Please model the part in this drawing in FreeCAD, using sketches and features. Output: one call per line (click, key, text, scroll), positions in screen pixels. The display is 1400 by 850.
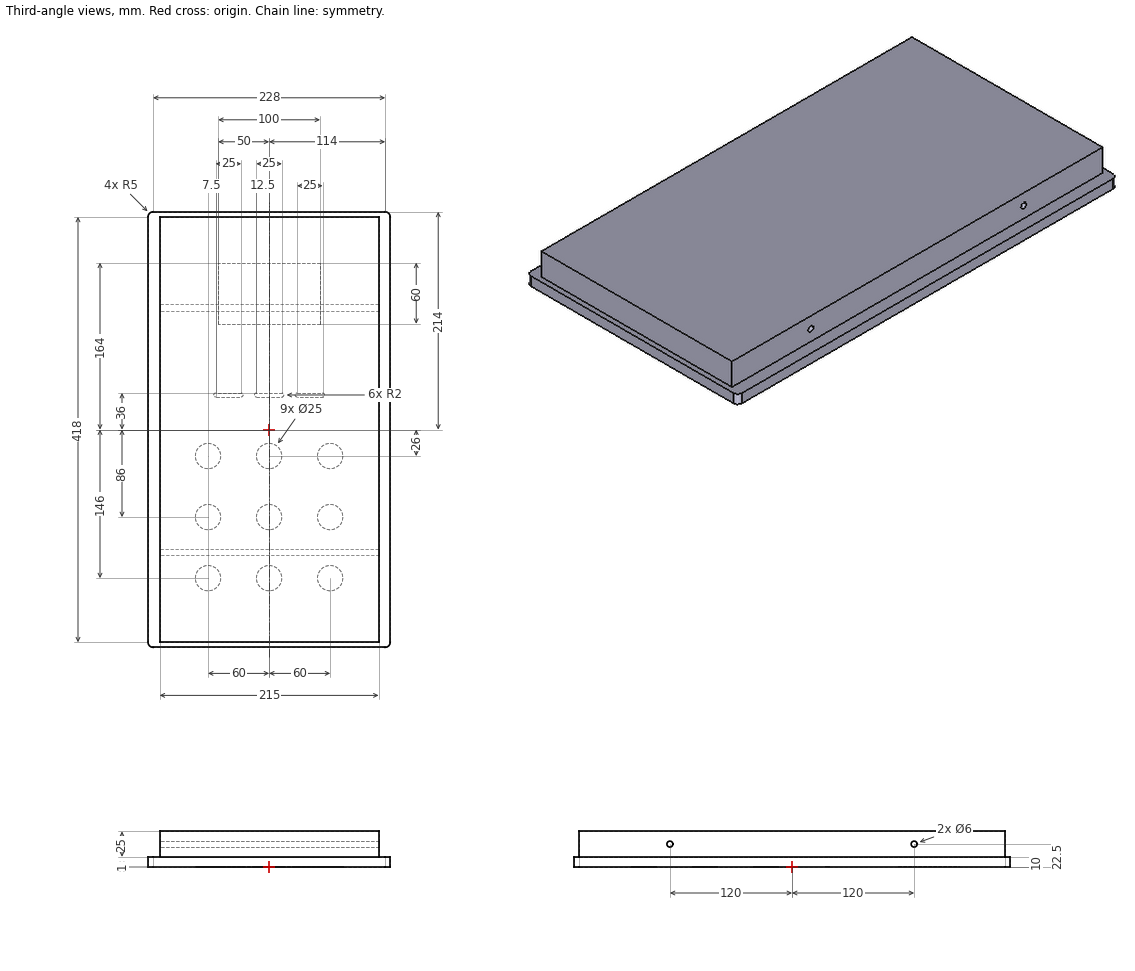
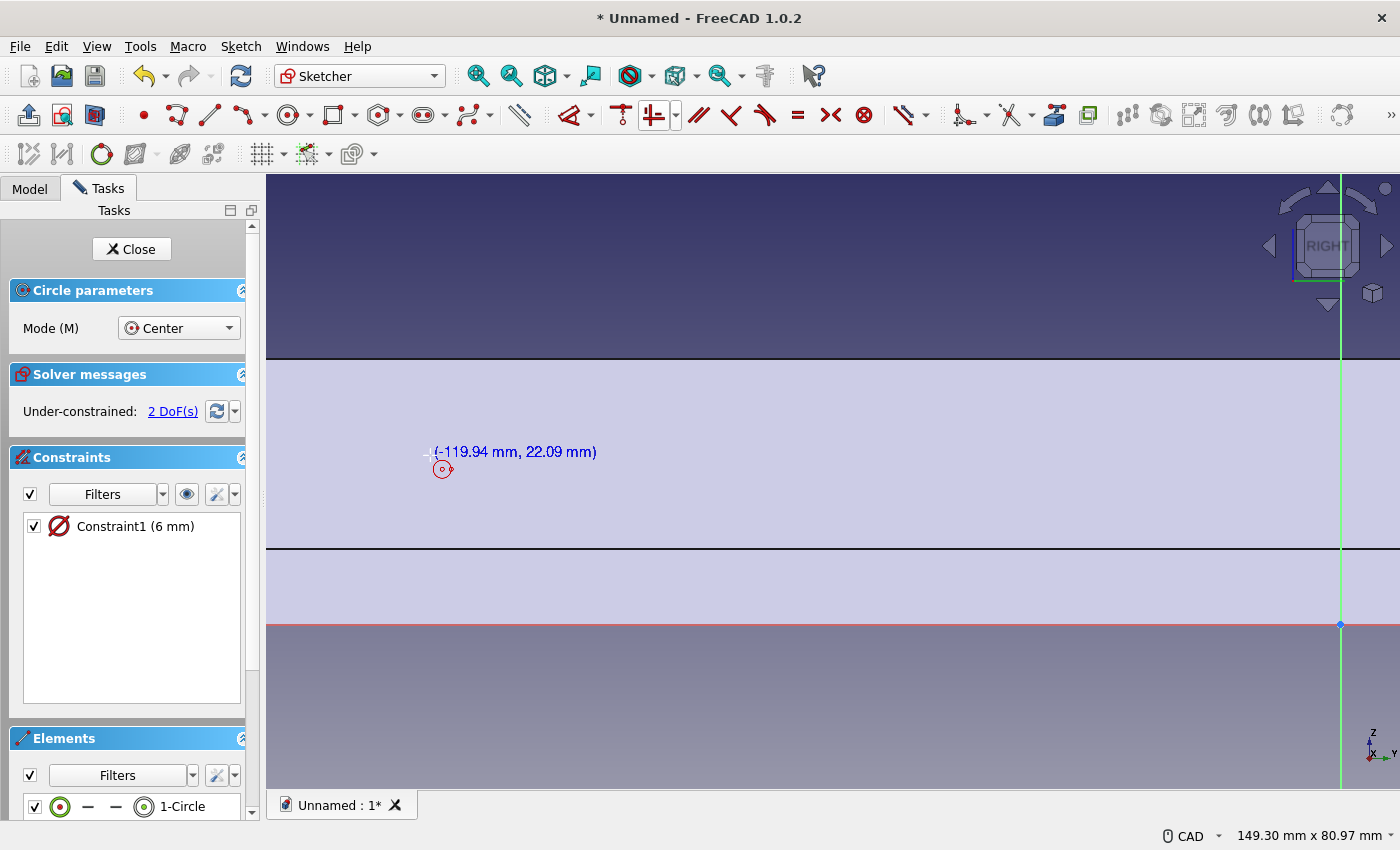
click(429, 454)
move(445, 438)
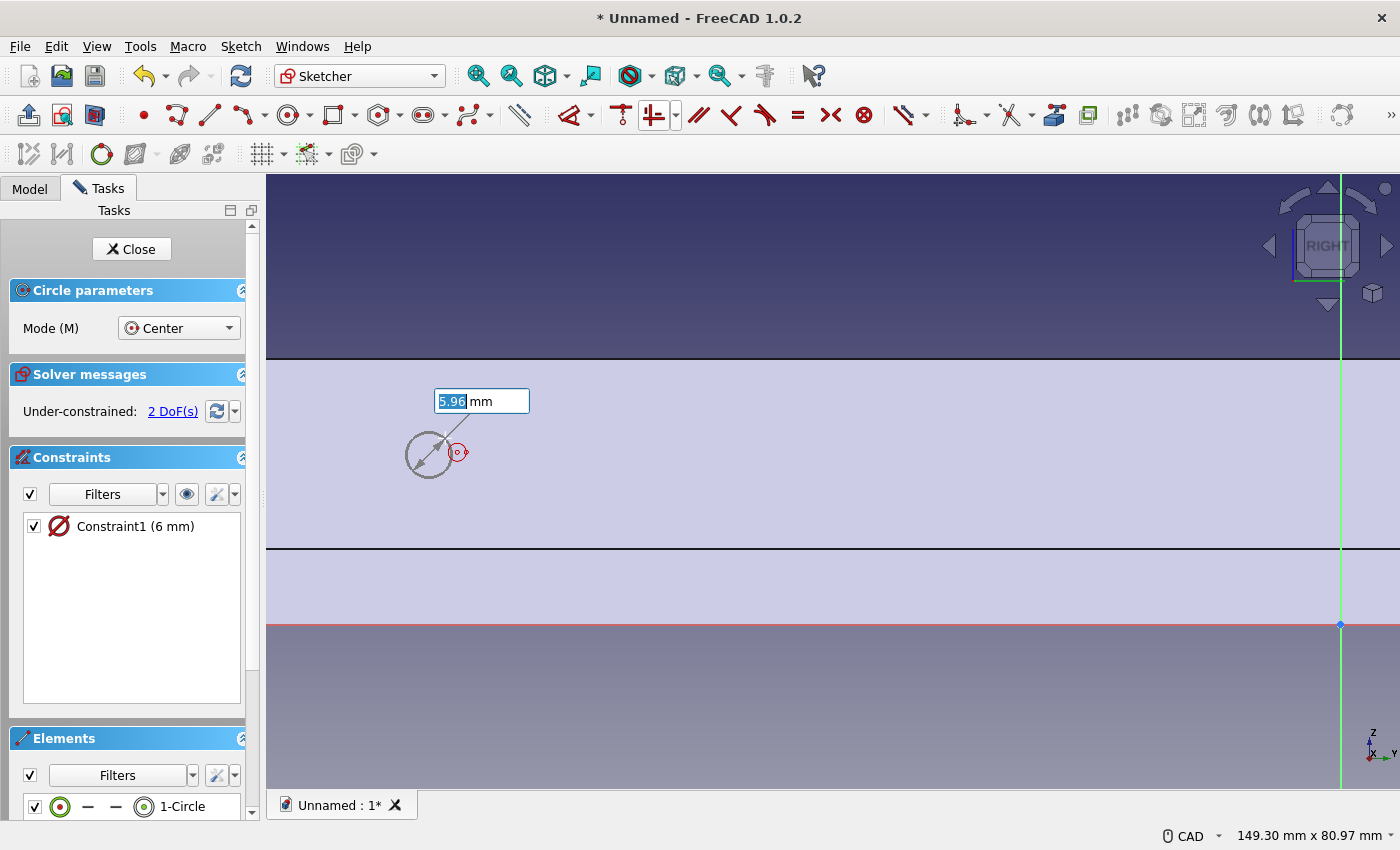
text(6)
key(Return)
key(Escape)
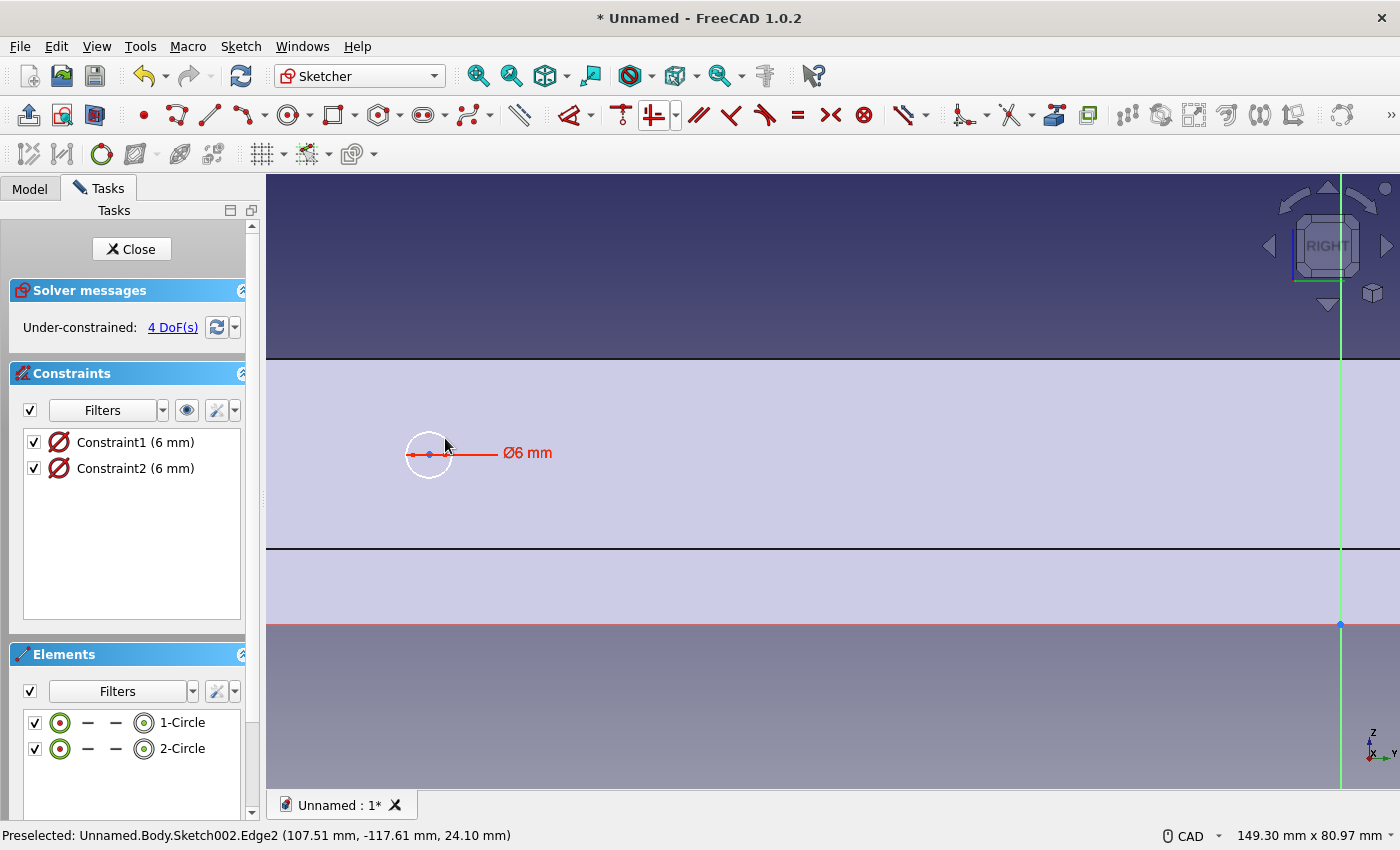
scroll(429, 455, down, 5)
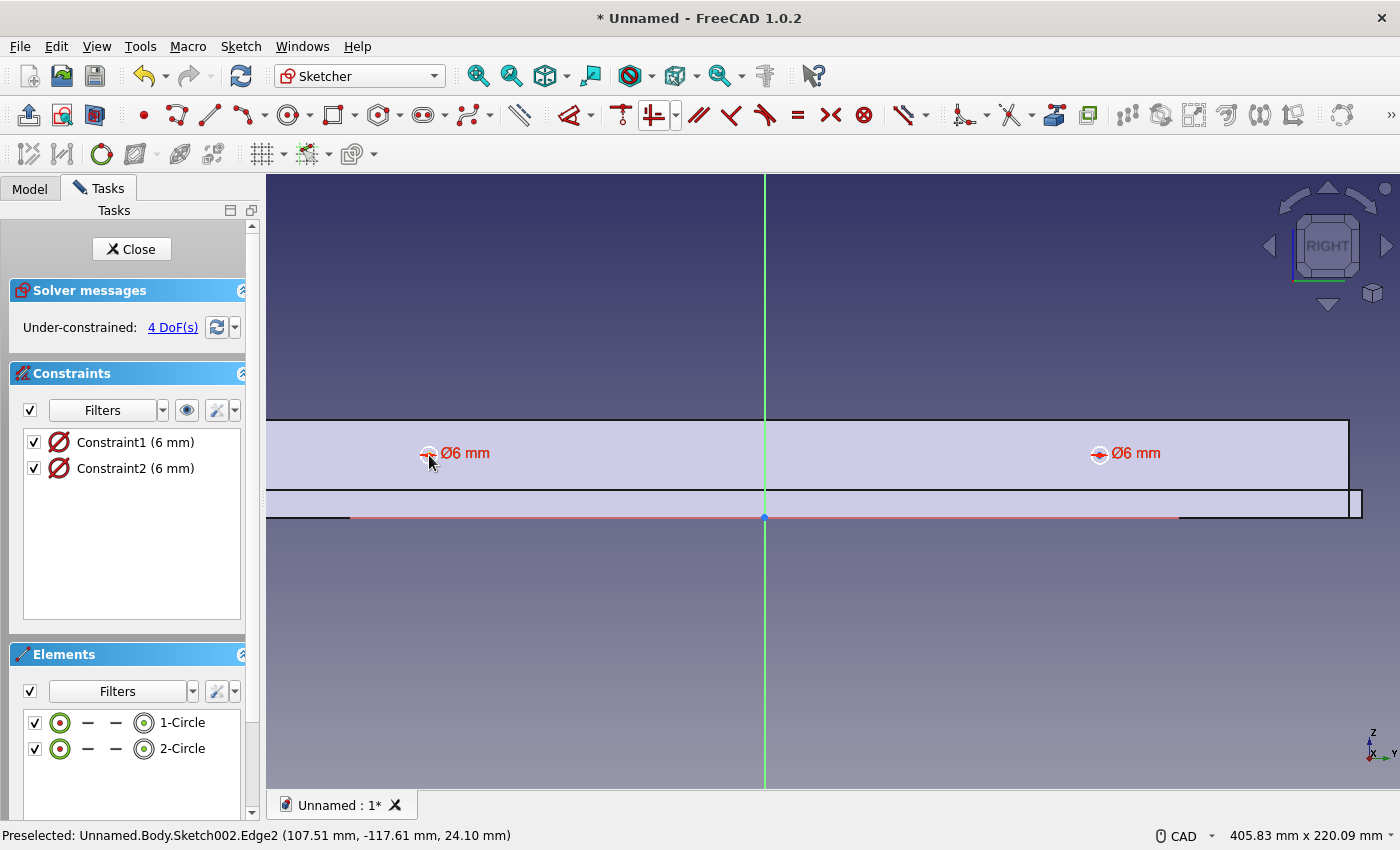
click(1100, 455)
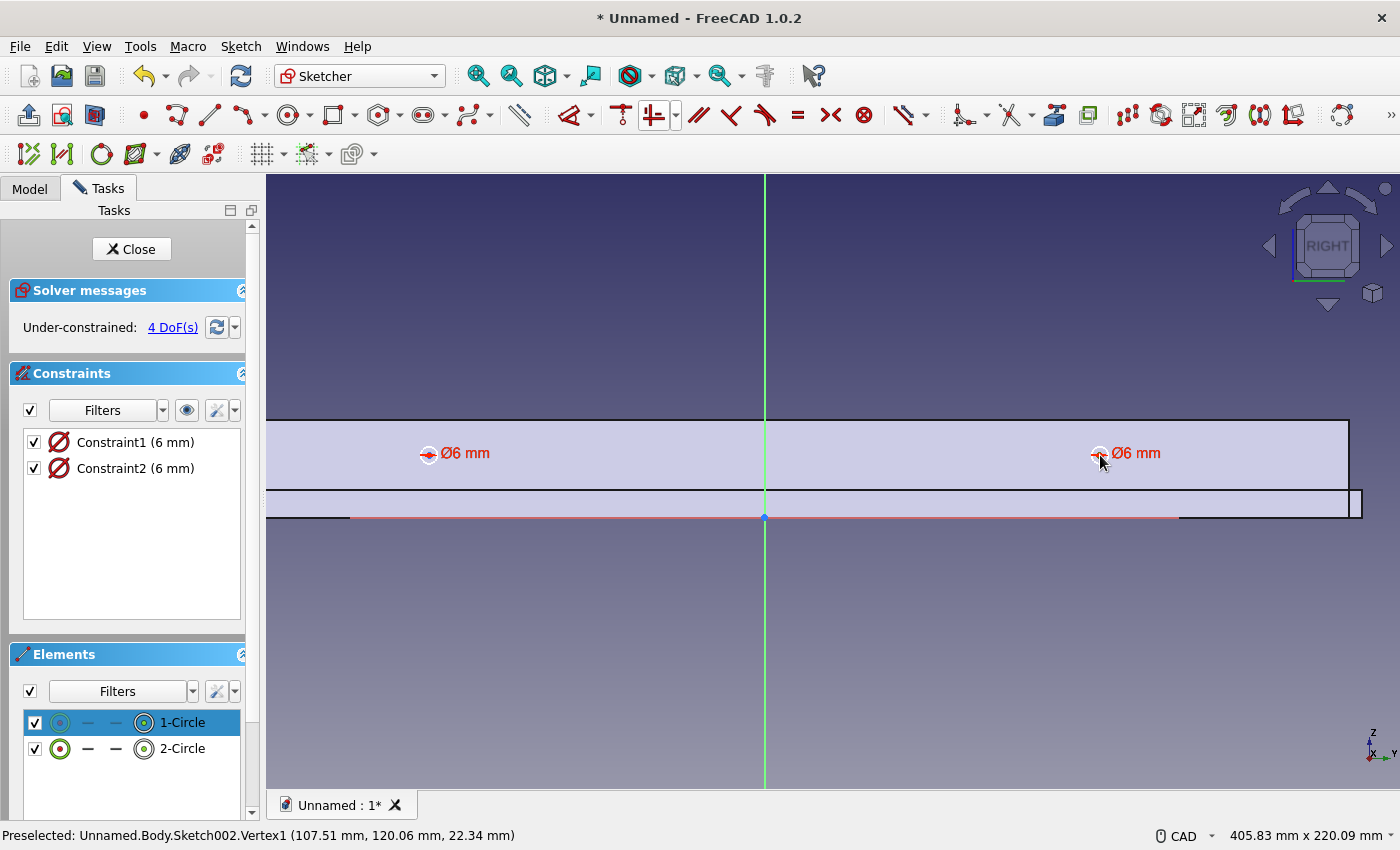
click(429, 455)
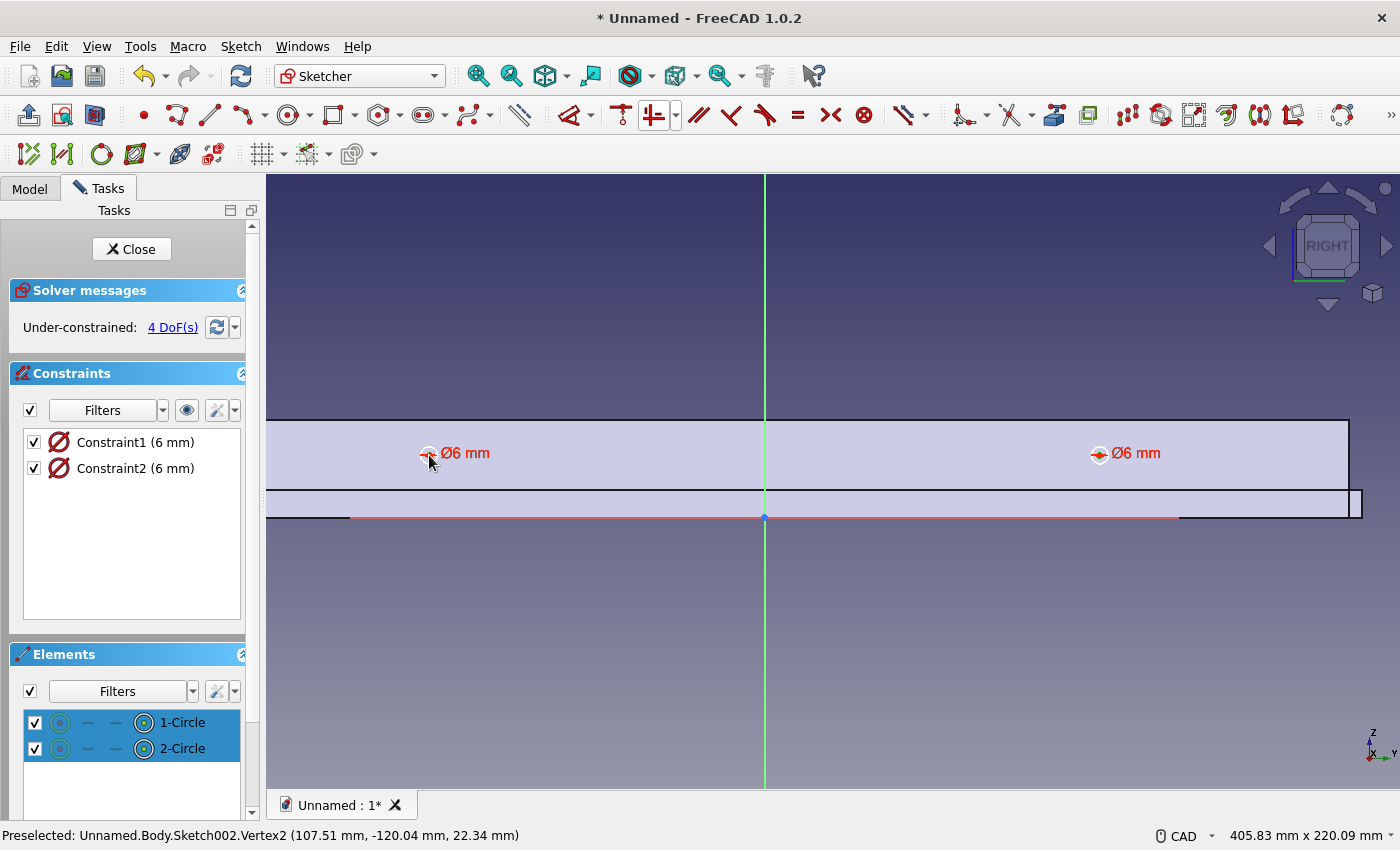
key(h)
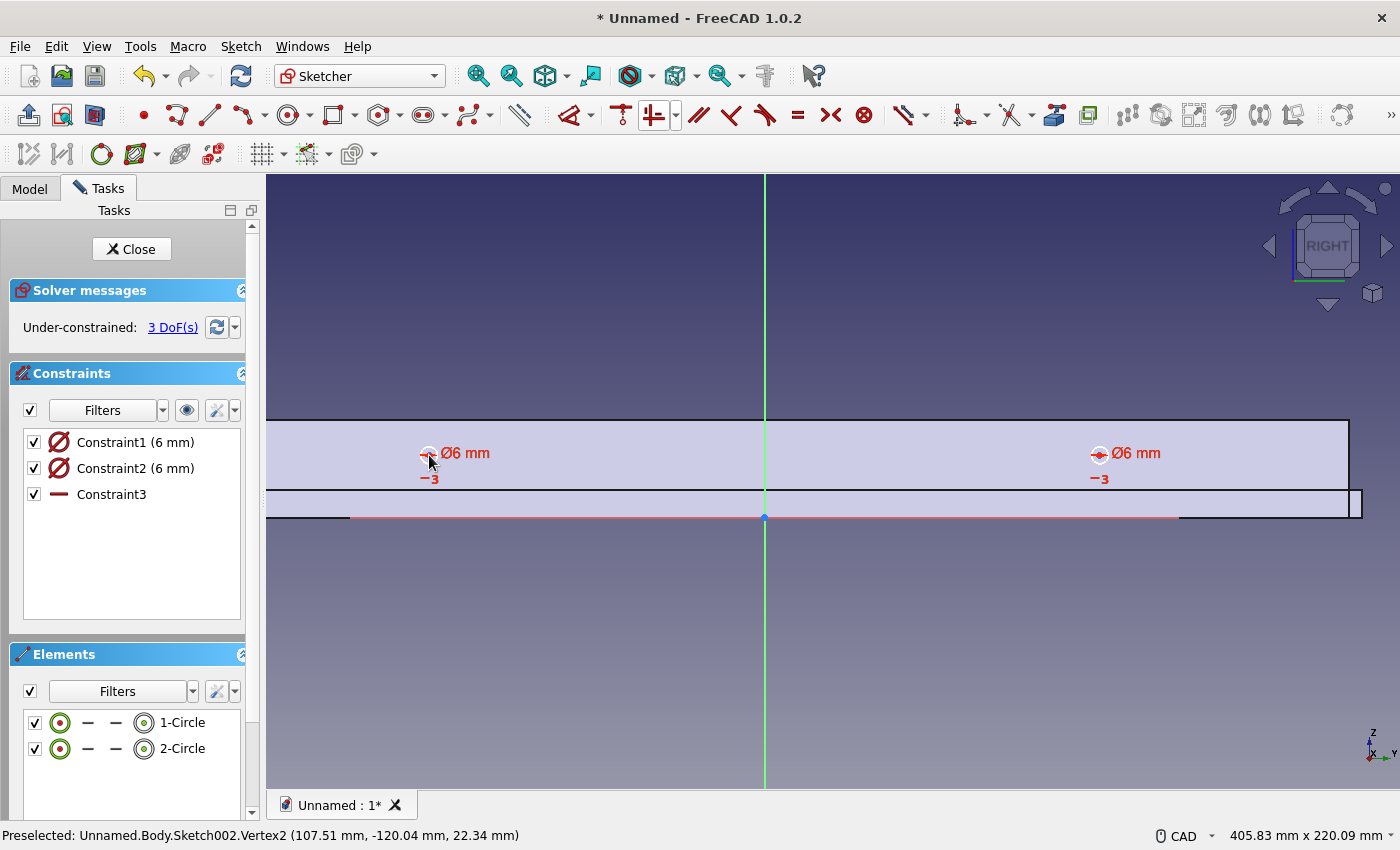
click(568, 116)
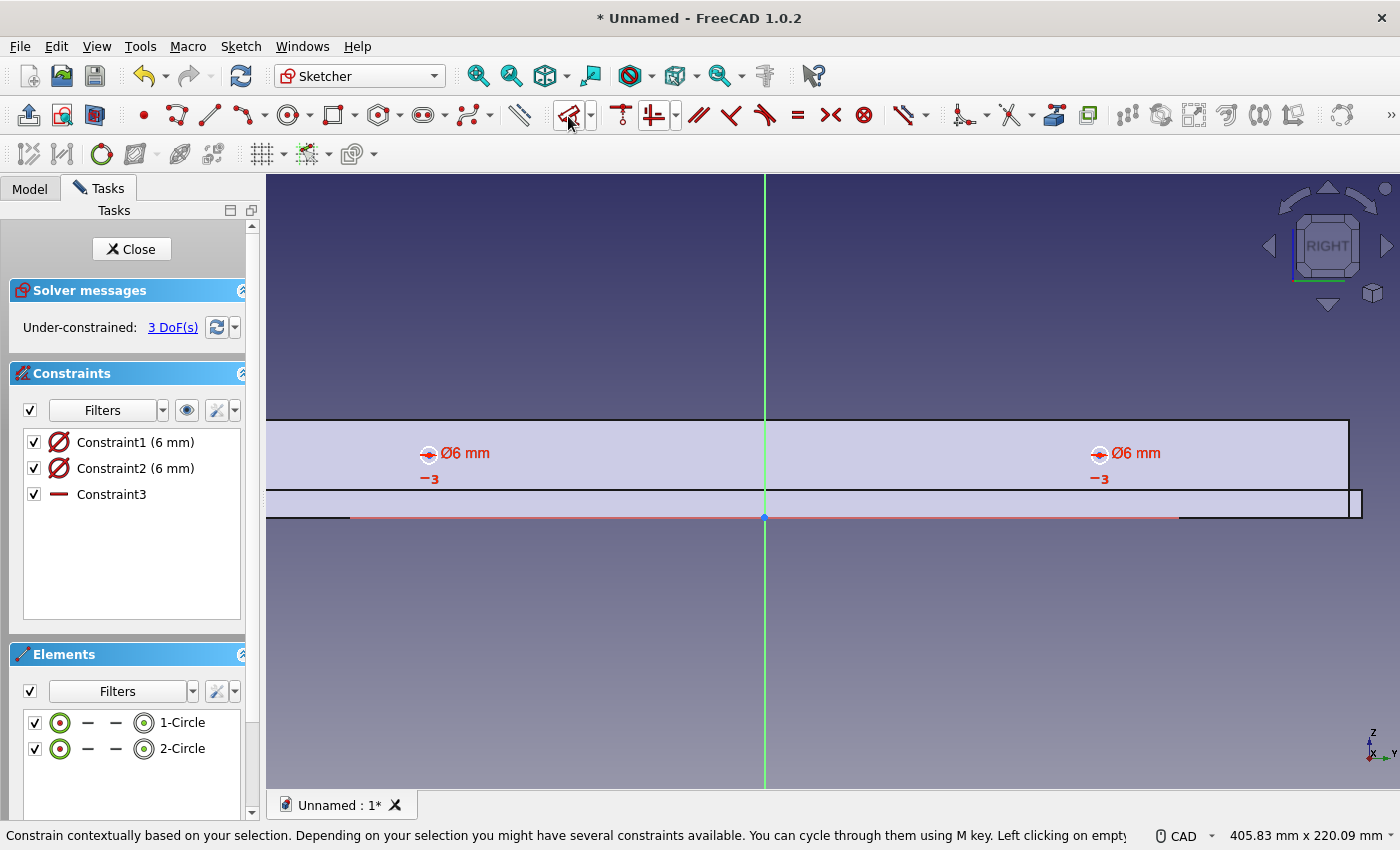
click(1100, 455)
click(932, 552)